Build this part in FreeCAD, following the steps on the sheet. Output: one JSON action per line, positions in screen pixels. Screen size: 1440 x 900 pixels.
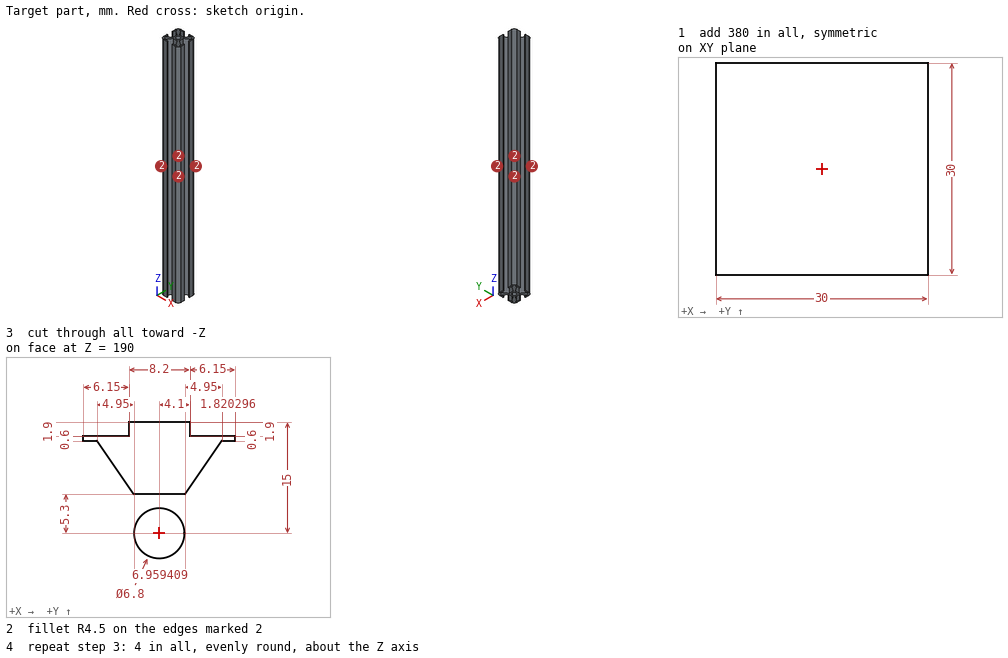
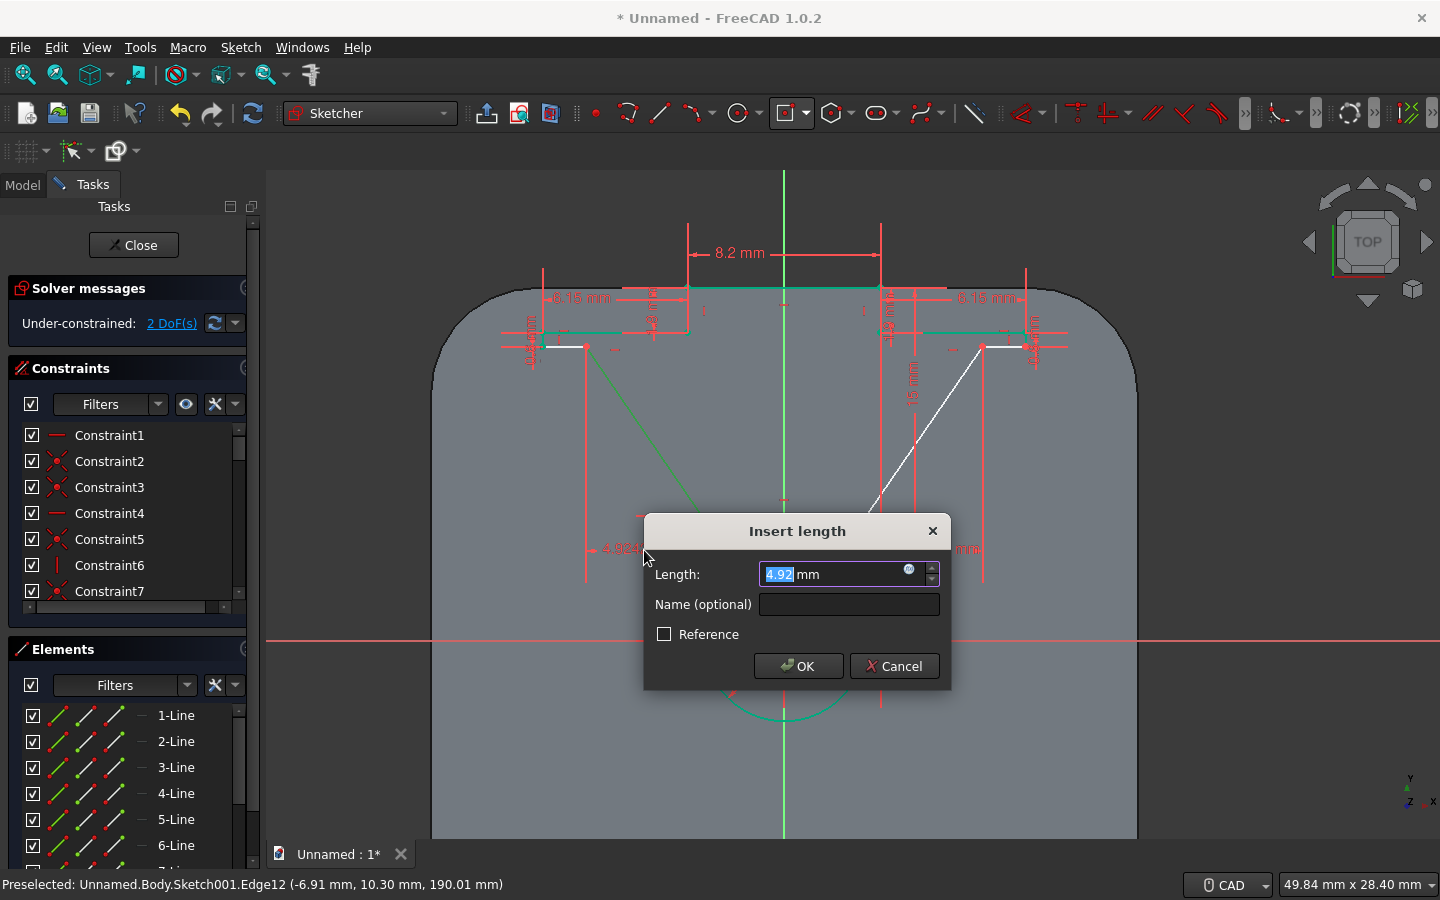
{"action": "type", "text": "4.95"}
{"action": "key", "text": "Return"}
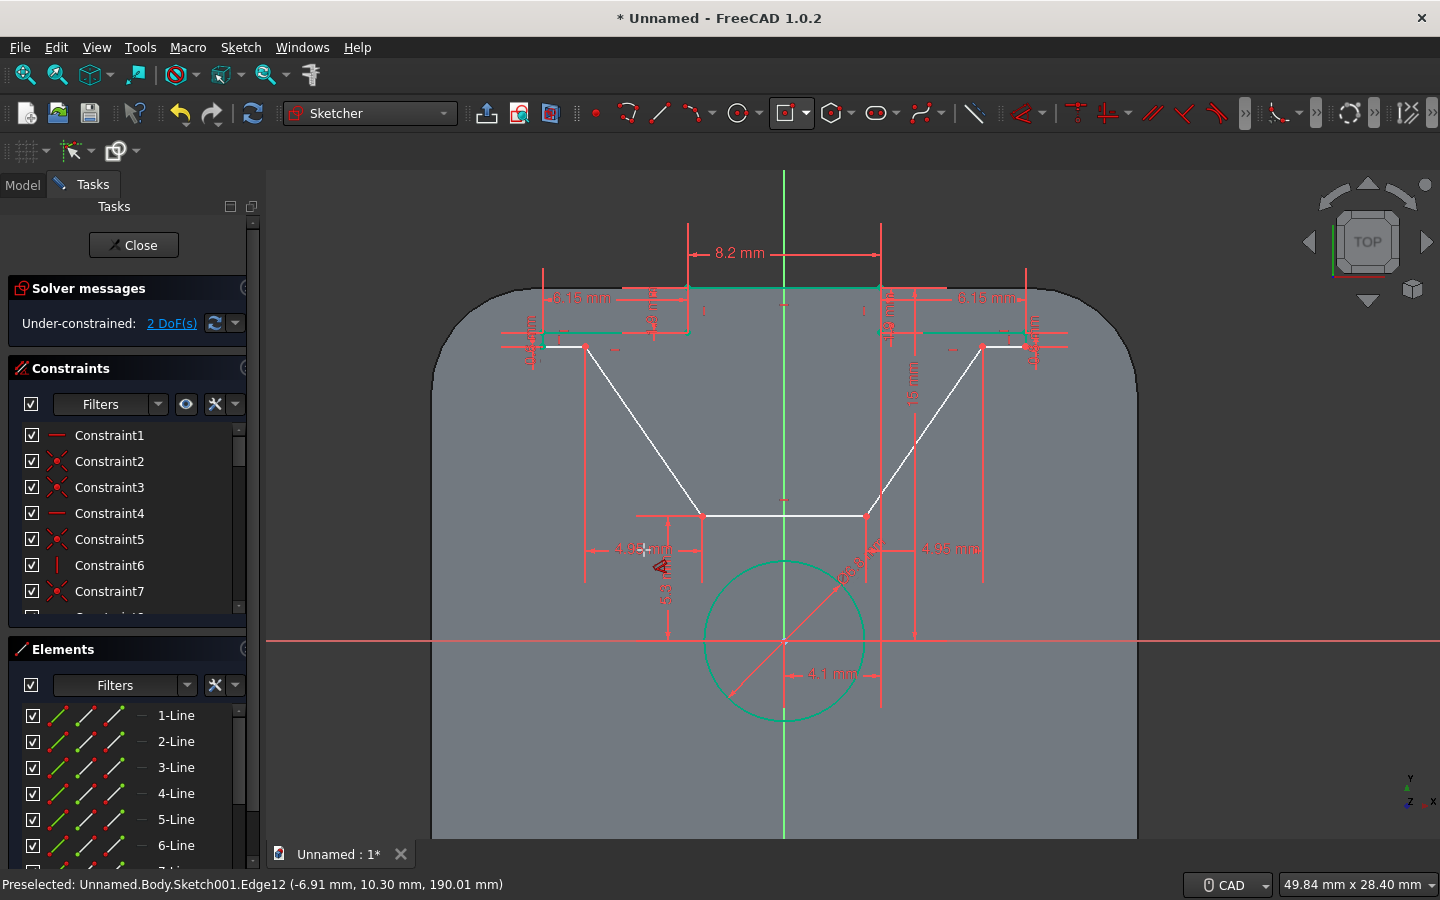
{"action": "left_click", "coordinate": [751, 516]}
{"action": "left_click", "coordinate": [746, 550]}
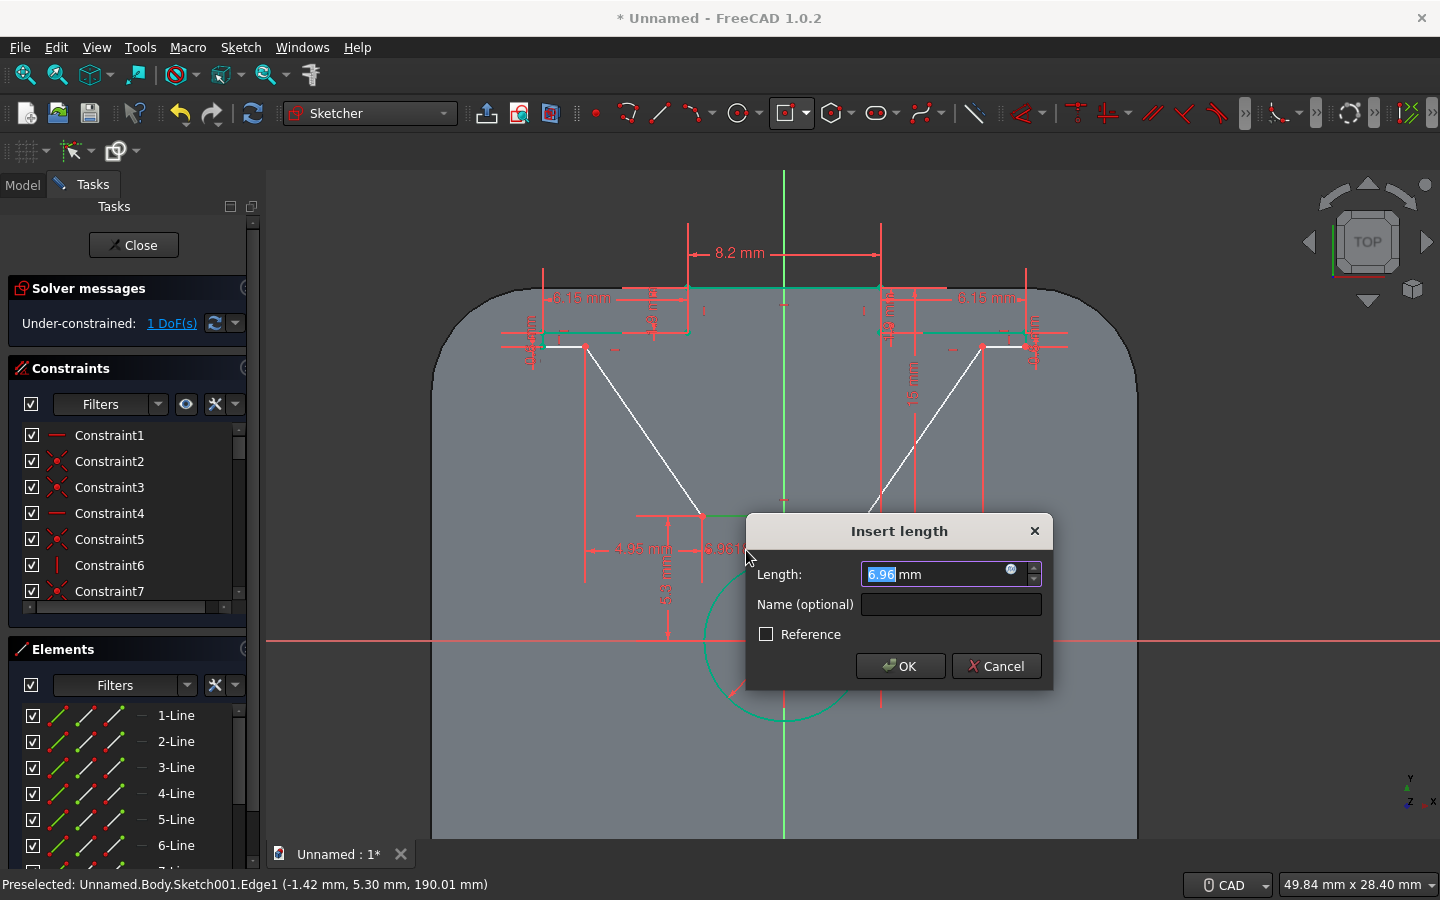
{"action": "type", "text": "6.959409"}
{"action": "key", "text": "Return"}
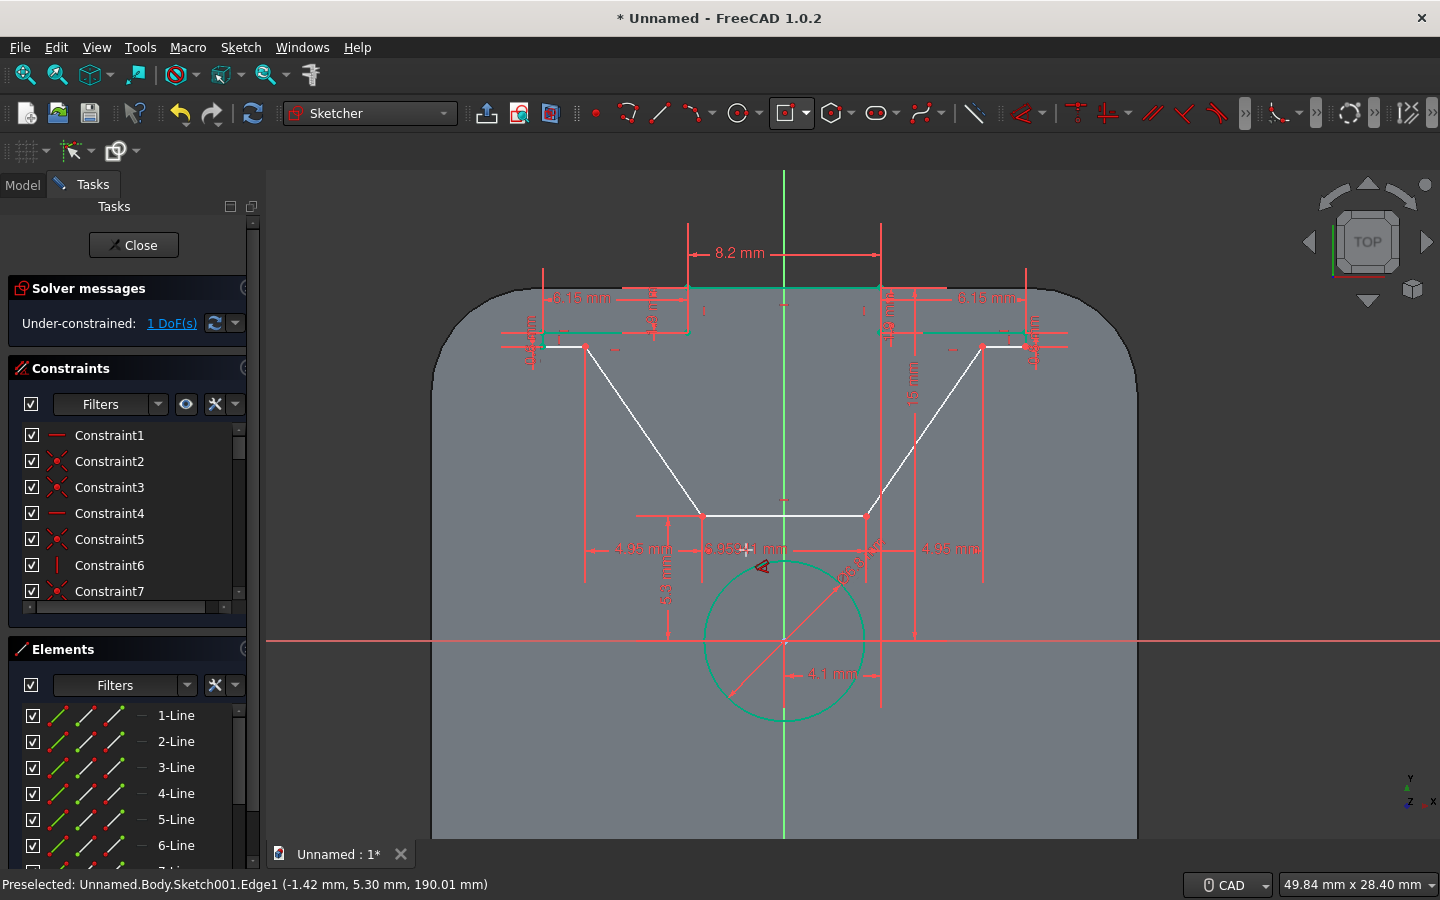
{"action": "left_click", "coordinate": [996, 347]}
{"action": "left_click", "coordinate": [1004, 381]}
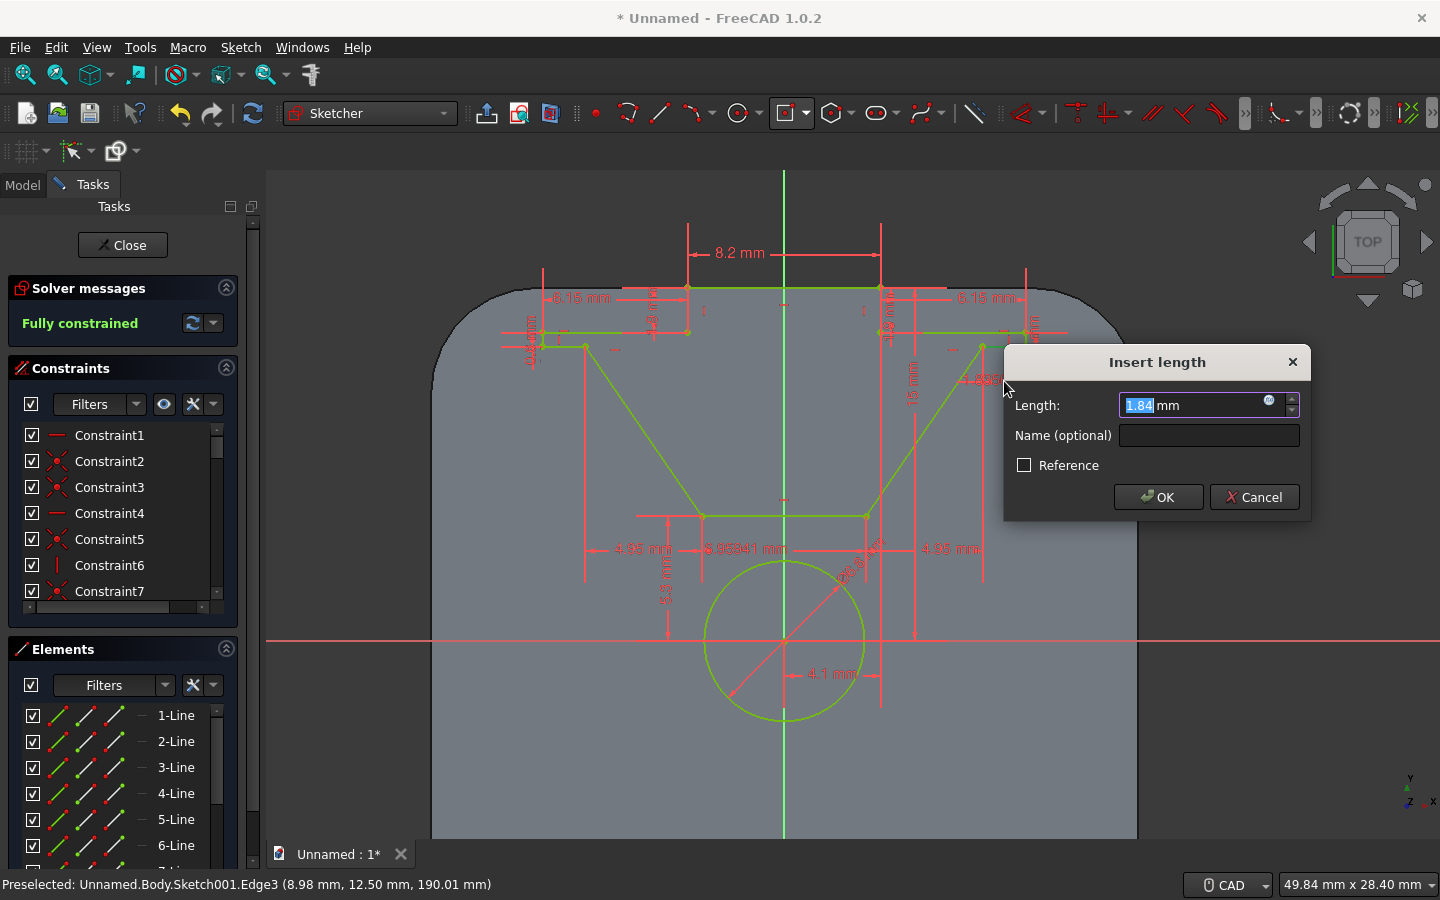
{"action": "type", "text": "1.820296"}
{"action": "key", "text": "Return"}
{"action": "key", "text": "Escape"}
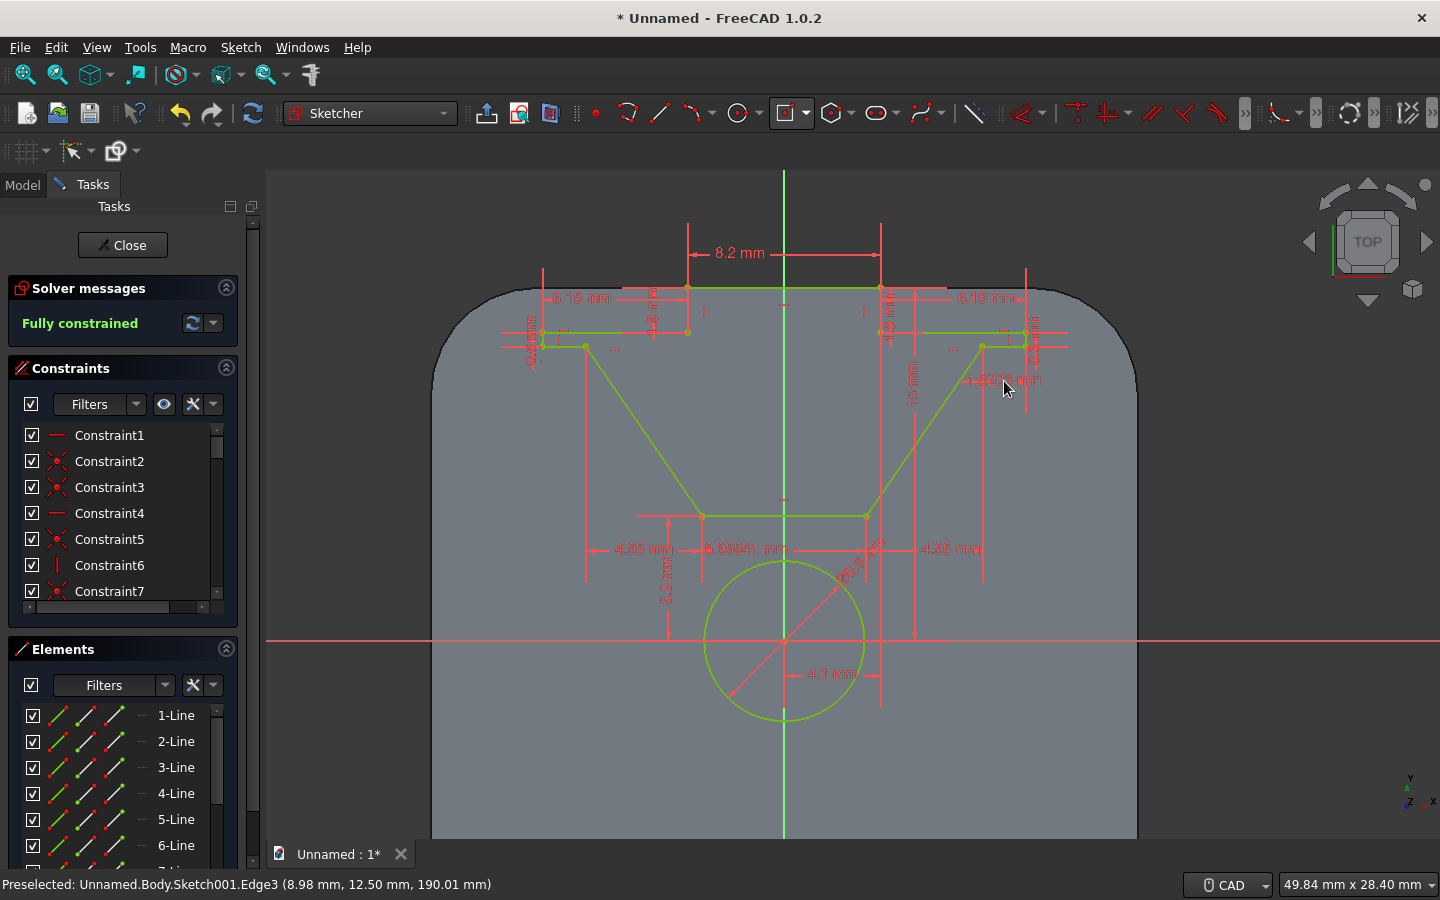
{"action": "left_click", "coordinate": [123, 245]}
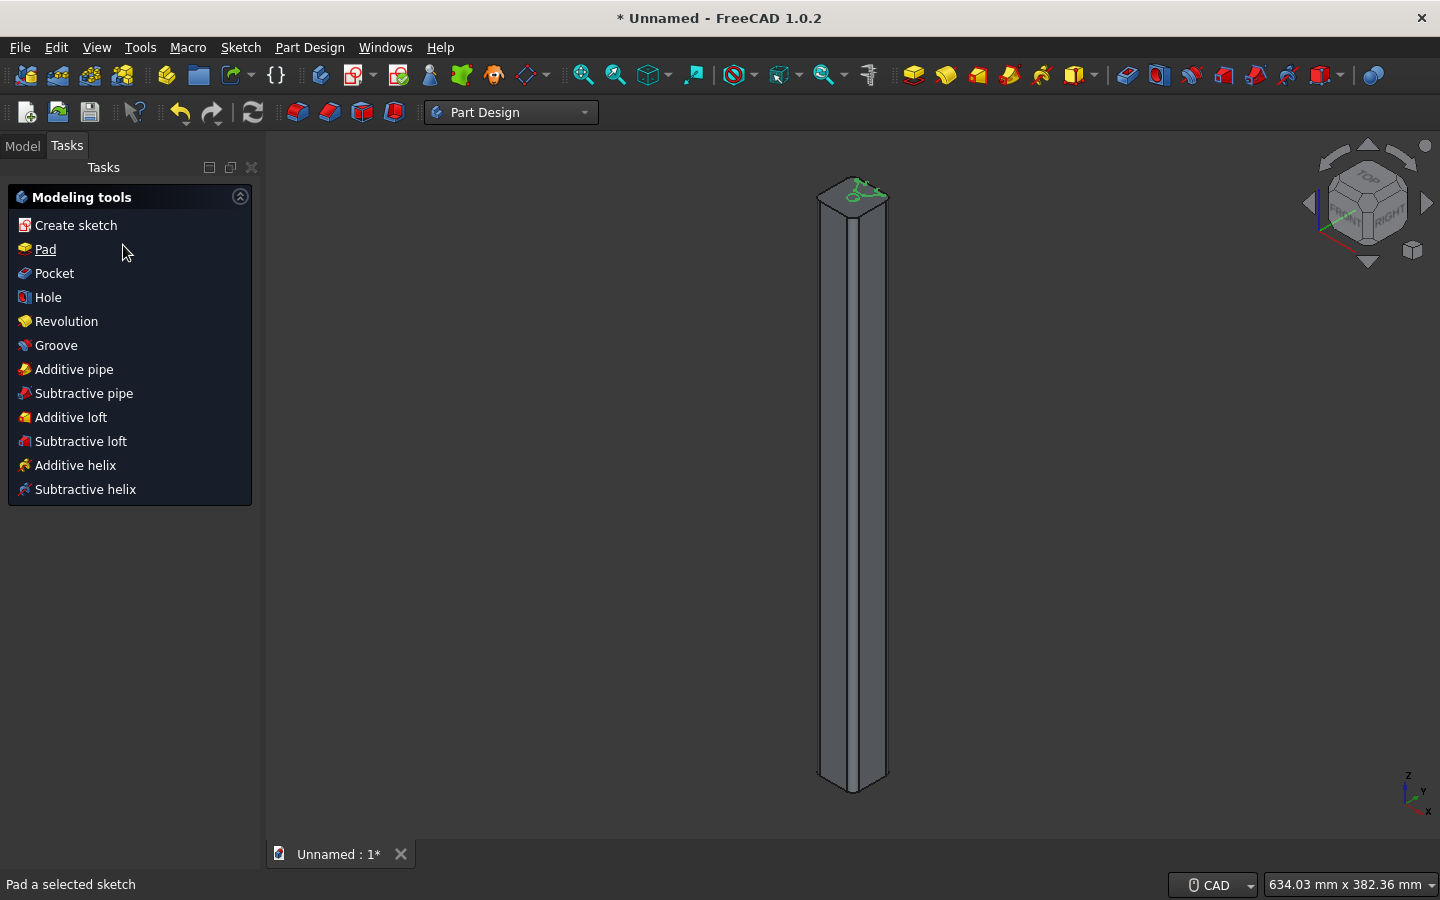
{"action": "left_click", "coordinate": [1128, 76]}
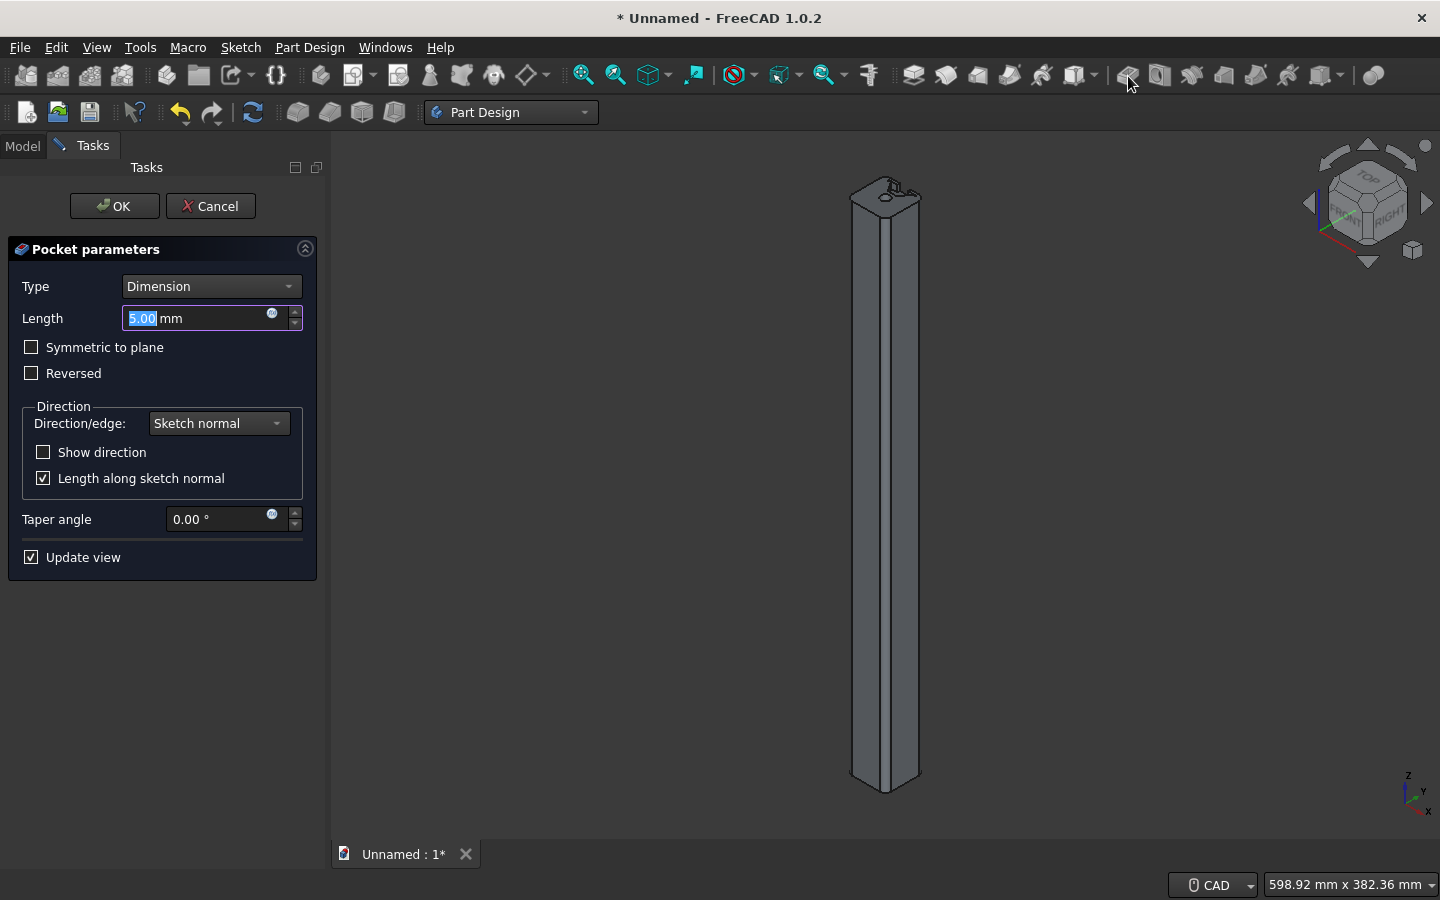
{"action": "left_click", "coordinate": [212, 286]}